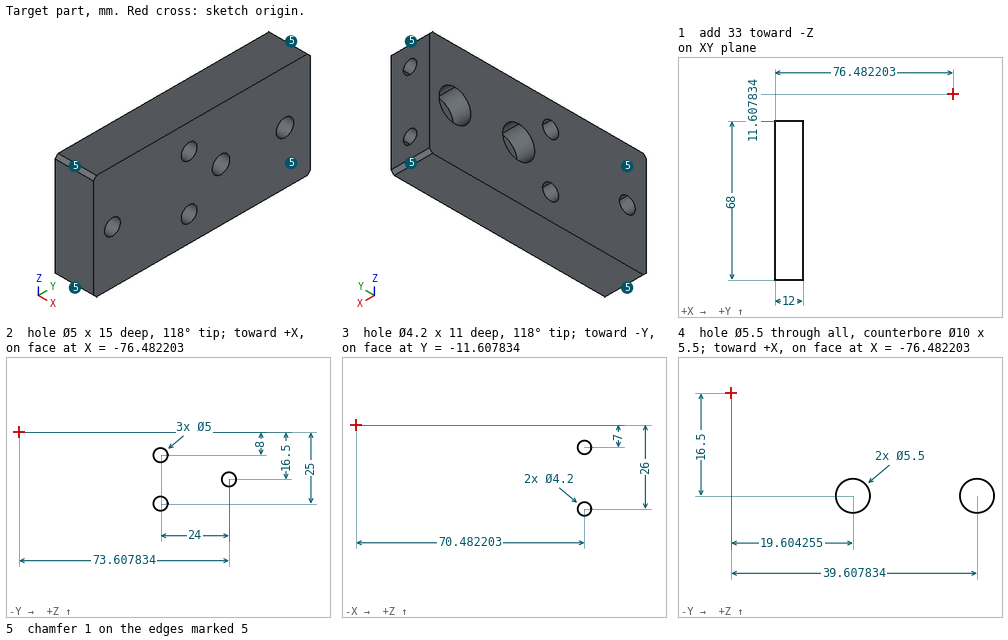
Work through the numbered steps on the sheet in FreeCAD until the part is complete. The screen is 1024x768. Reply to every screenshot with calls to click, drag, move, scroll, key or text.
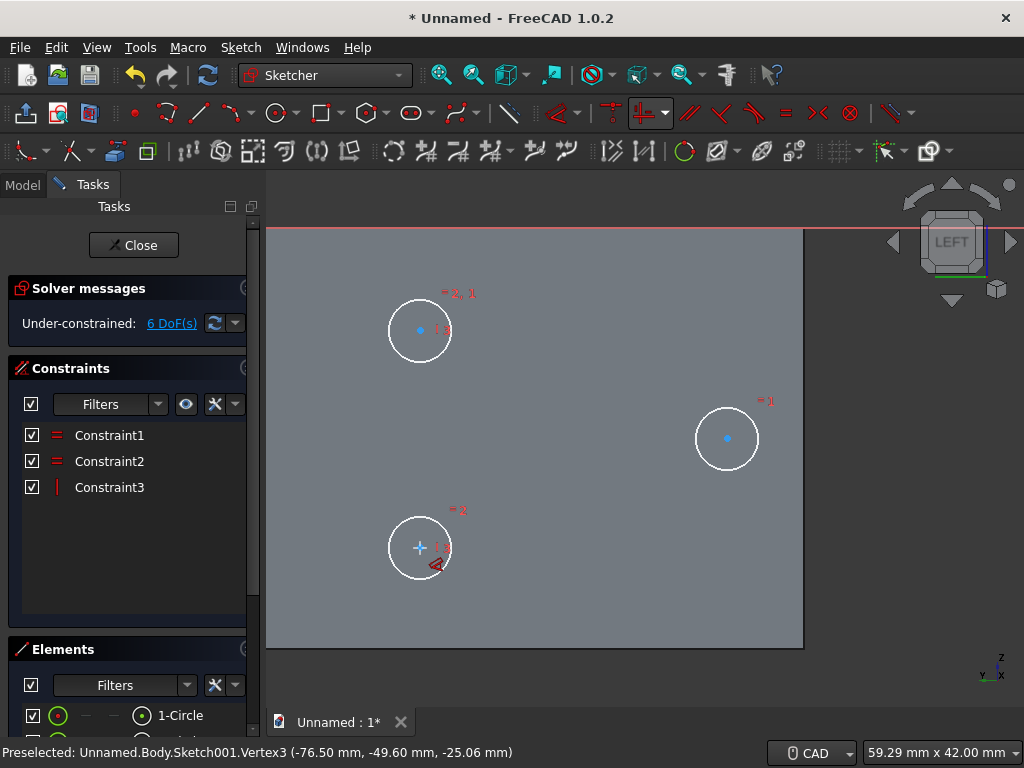
click(749, 417)
click(772, 394)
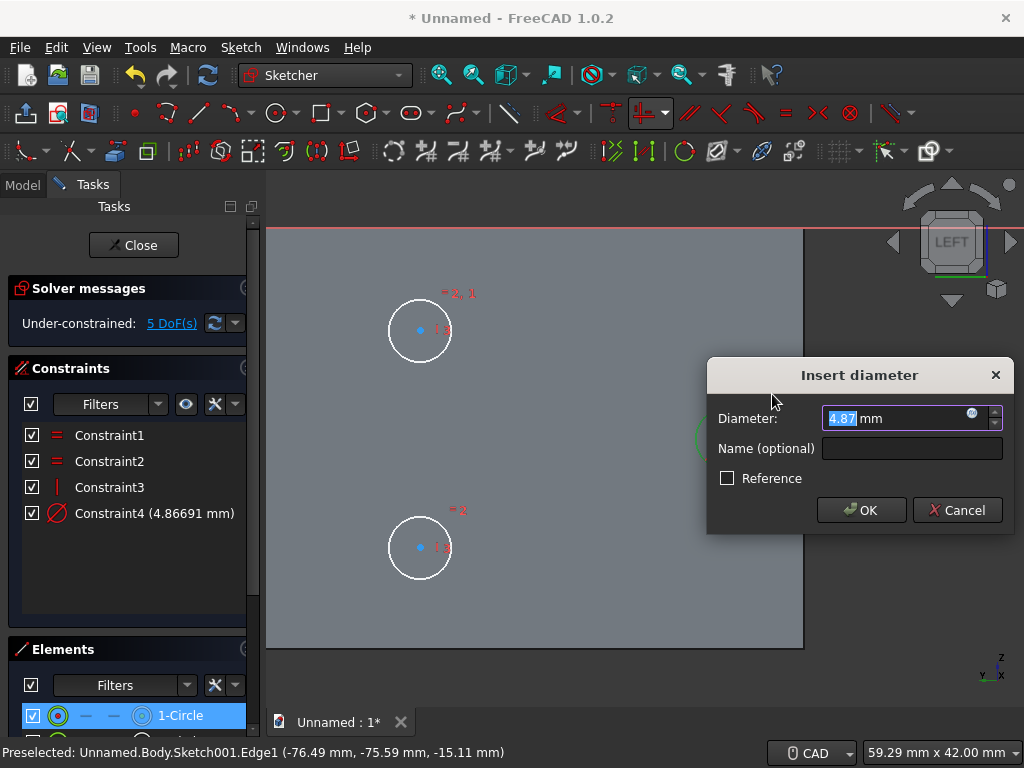
text(5)
key(Return)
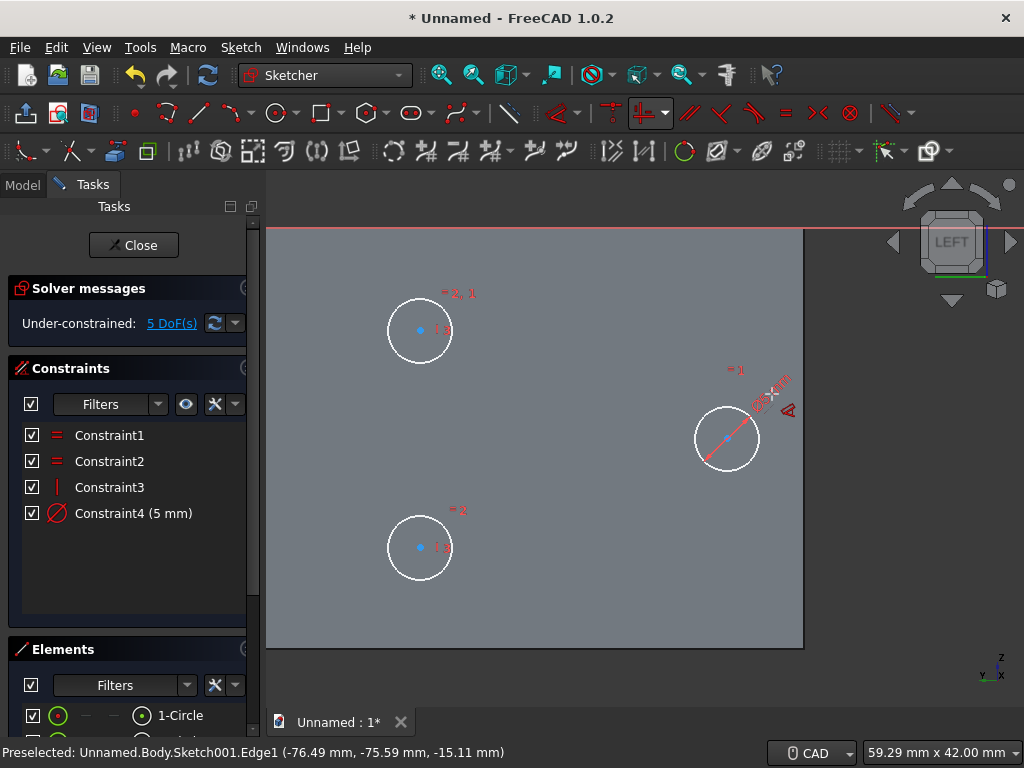
click(420, 331)
click(454, 279)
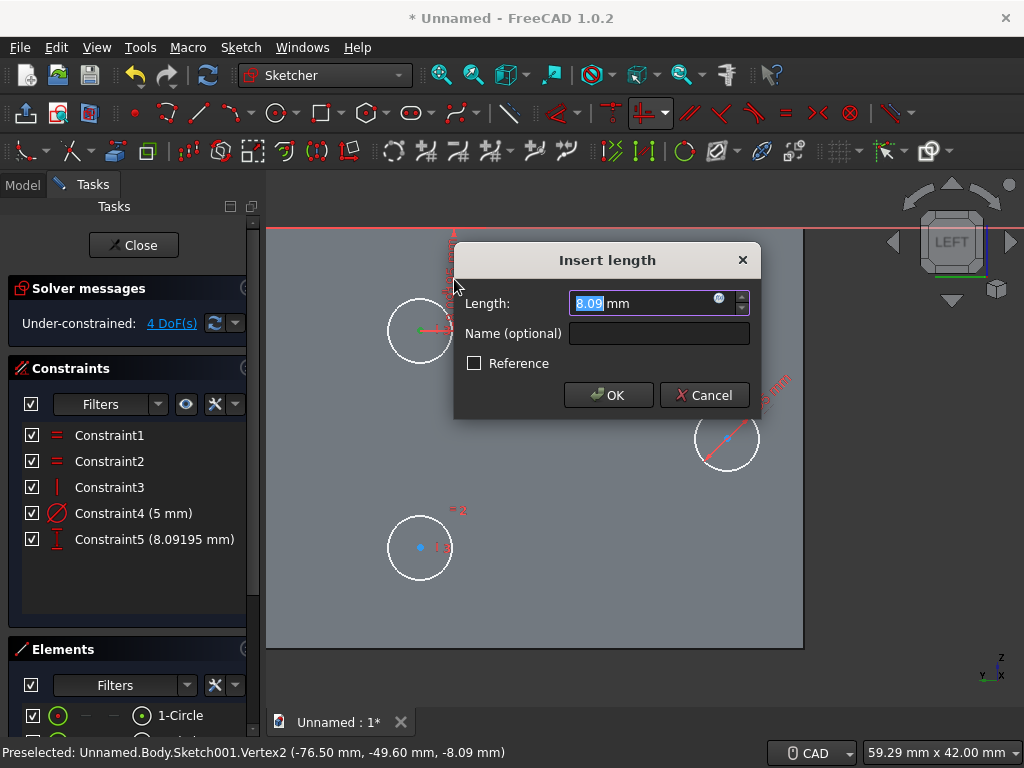
text(8)
key(Return)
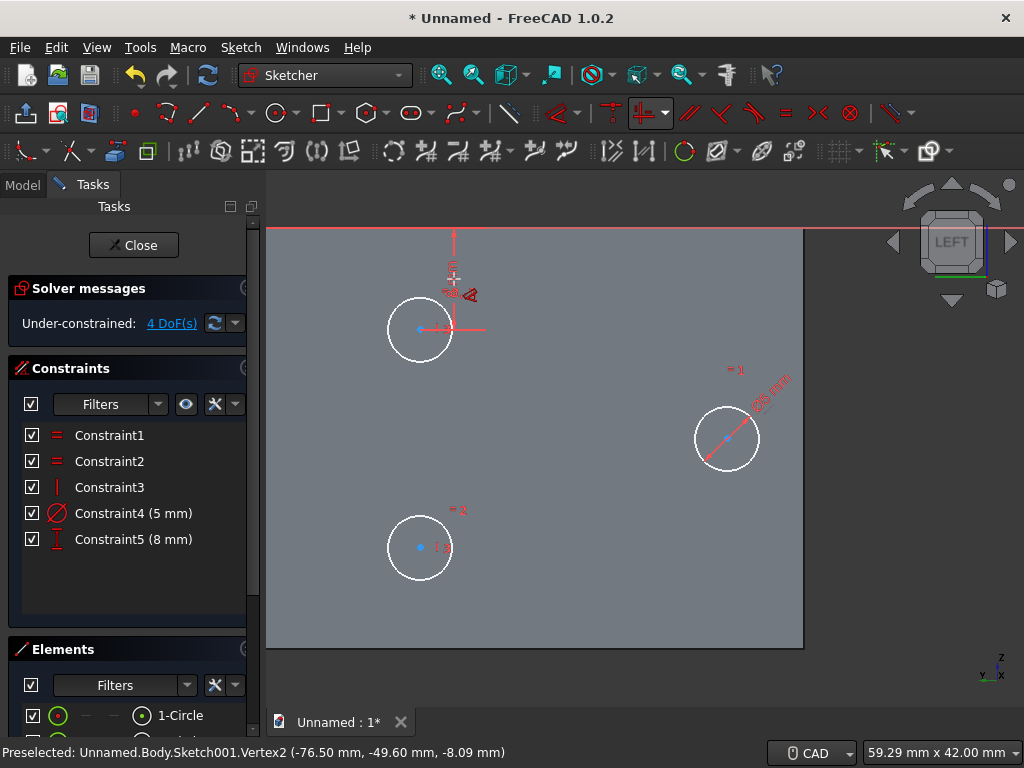
click(420, 548)
click(454, 388)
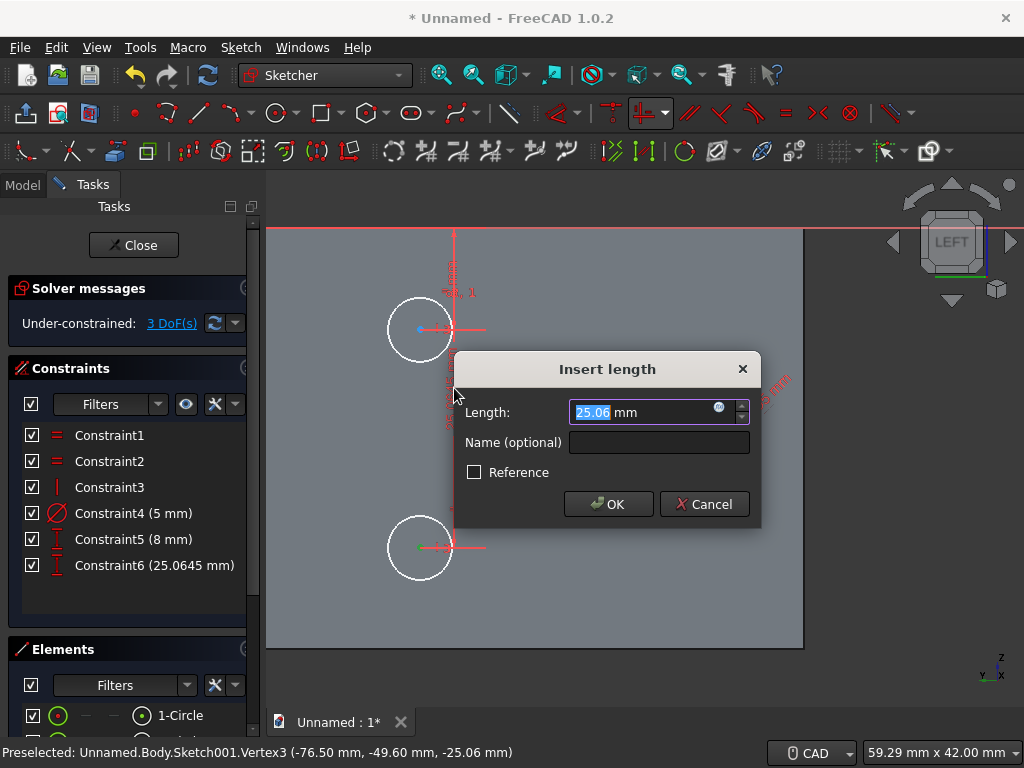
text(25)
key(Return)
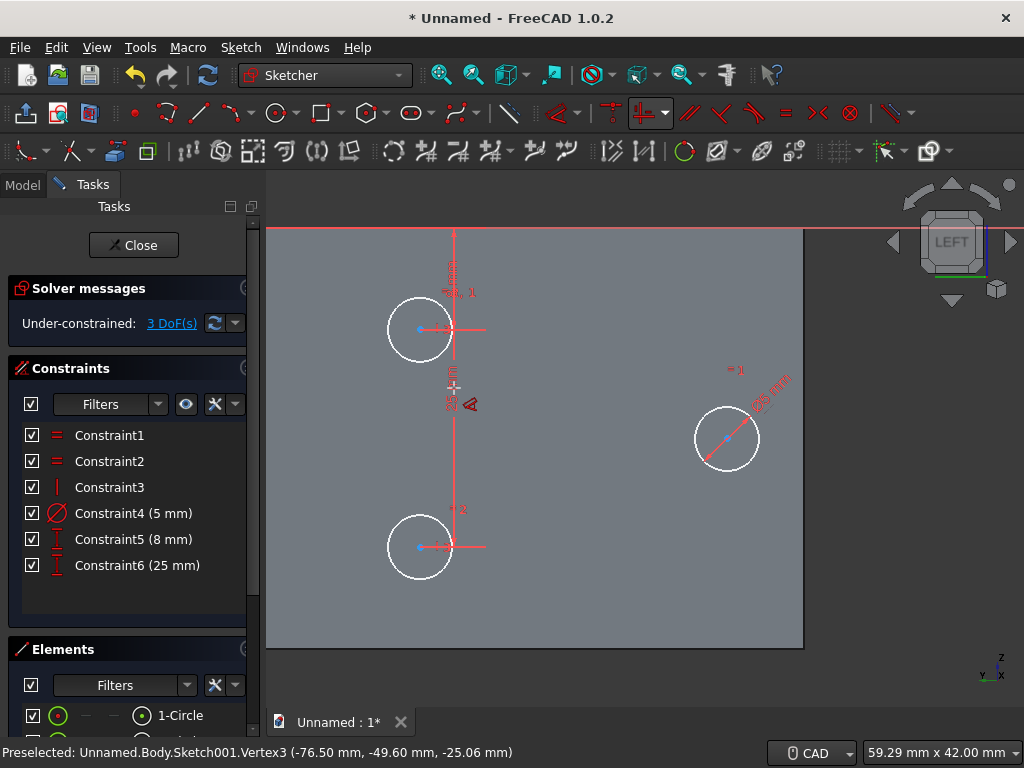
click(727, 439)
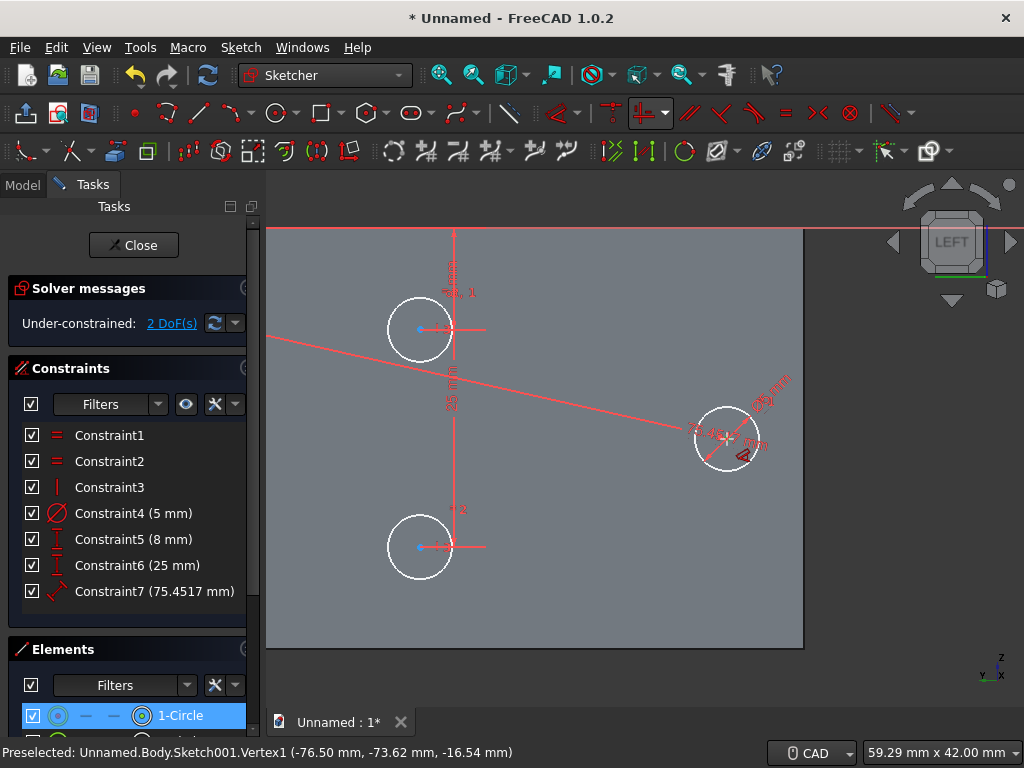
click(420, 330)
click(574, 296)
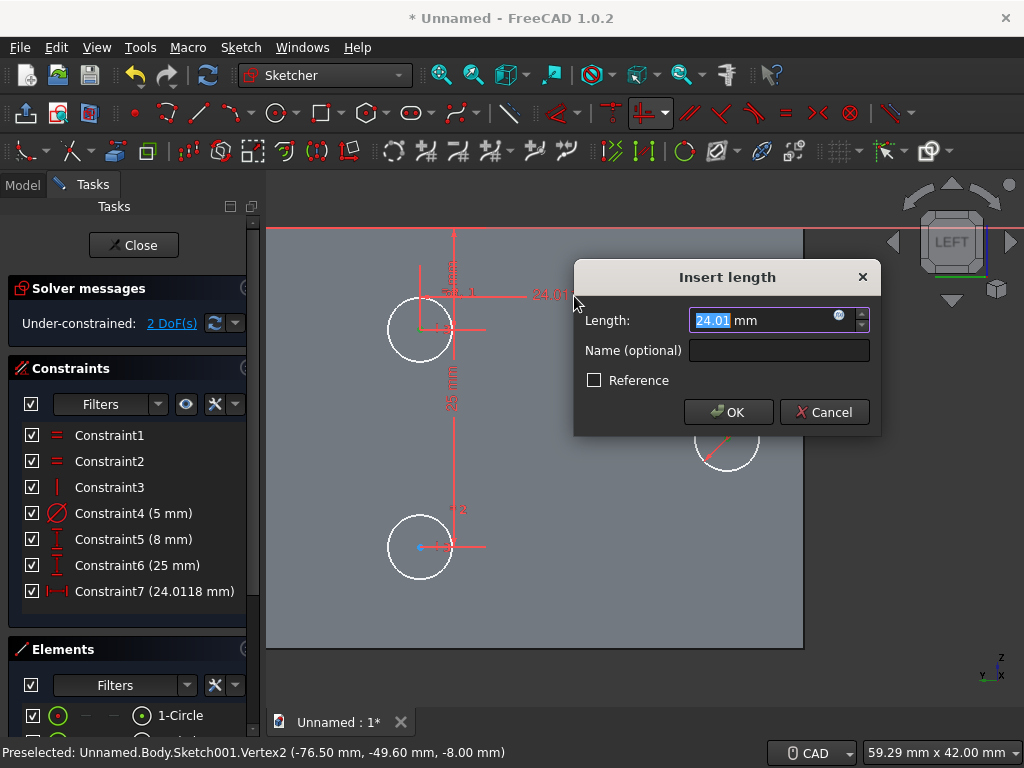
text(24)
key(Return)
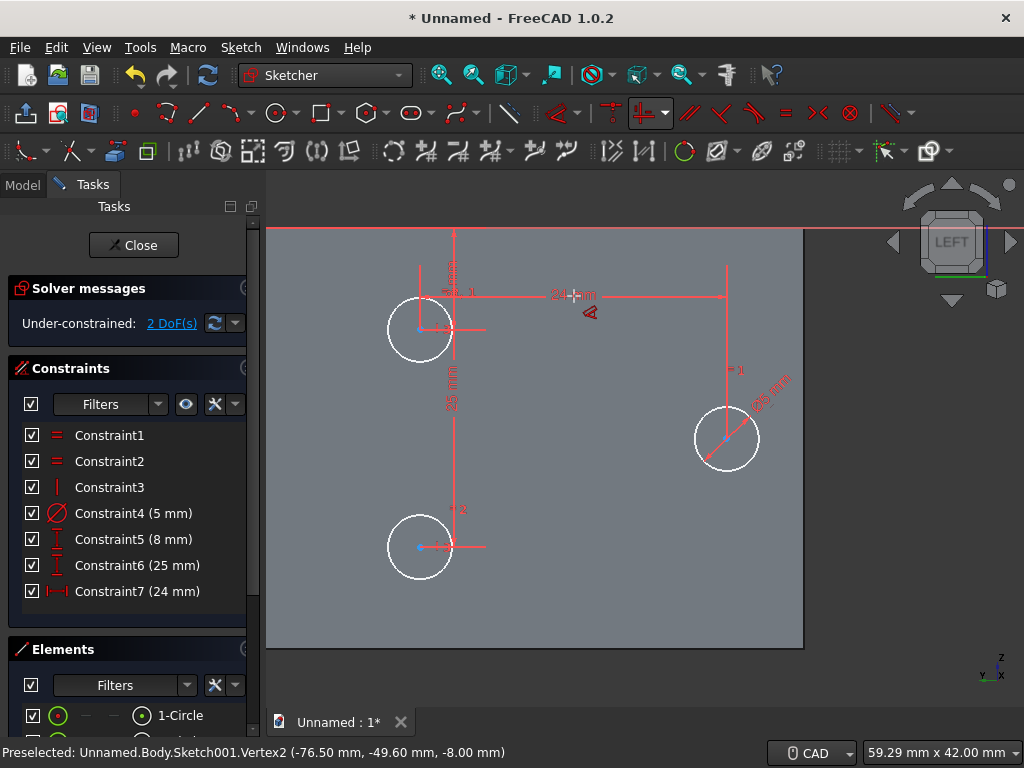
click(727, 439)
click(761, 333)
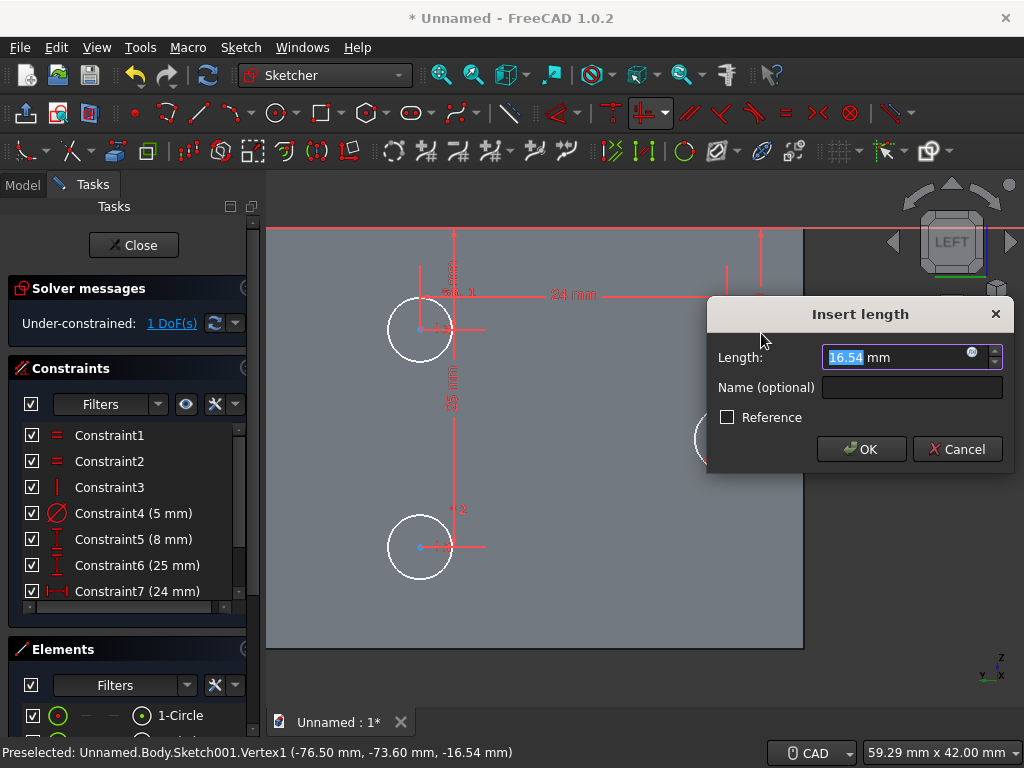
text(16.5)
key(Return)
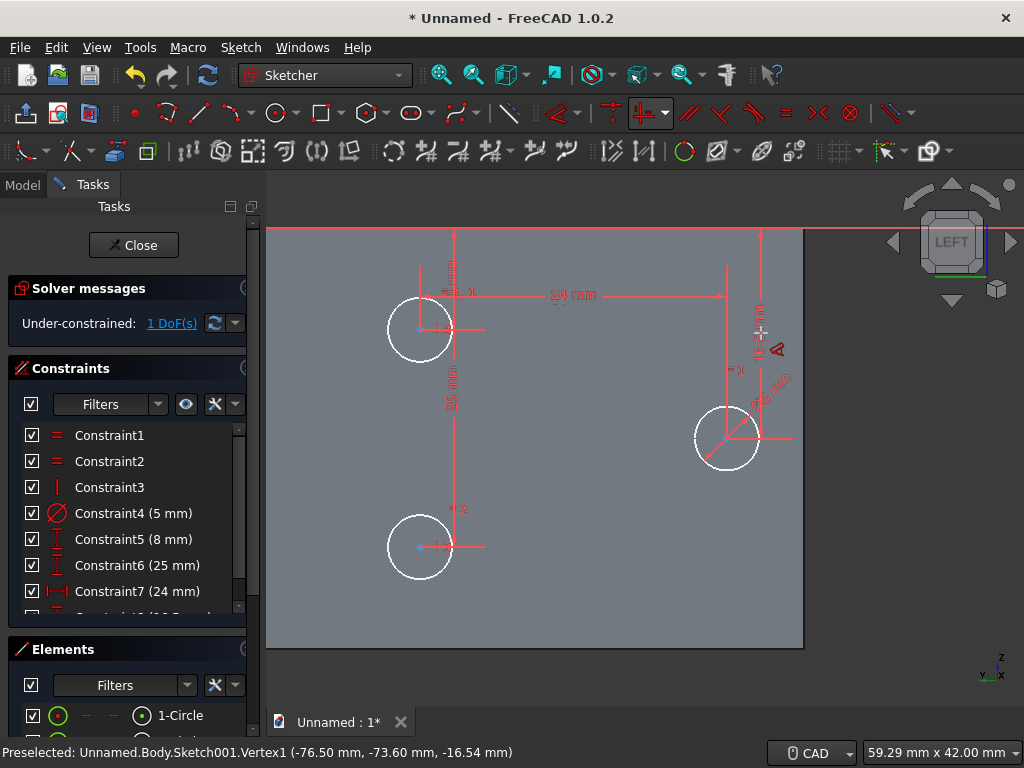
click(727, 438)
click(510, 472)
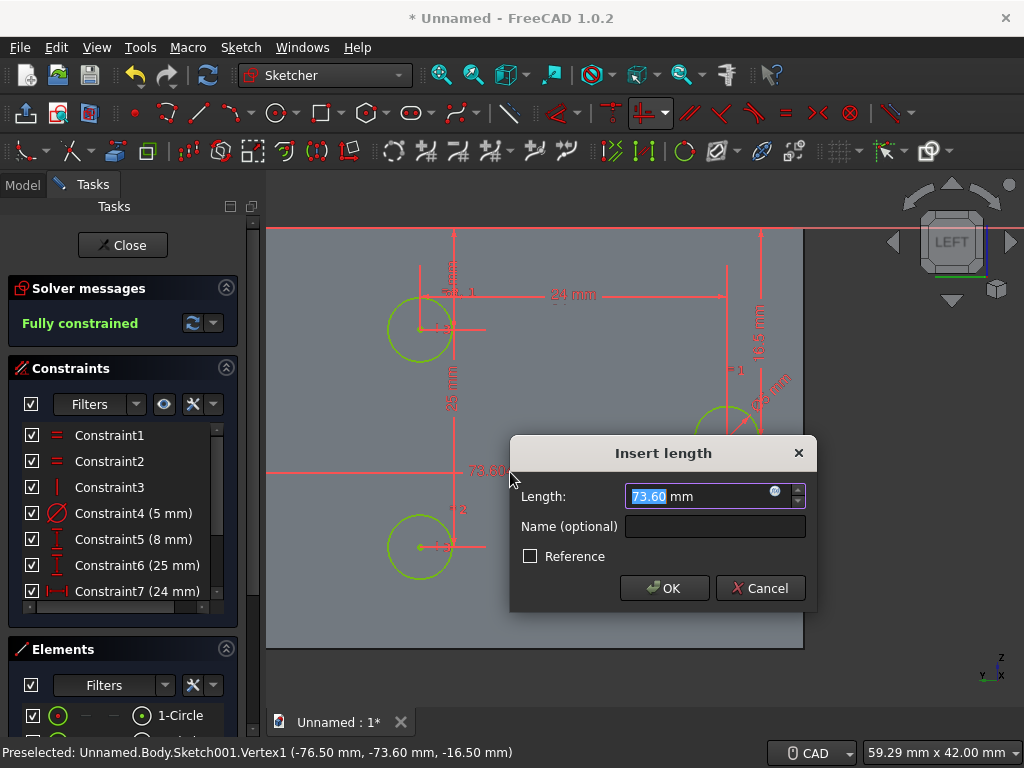
text(73.607834)
key(Return)
key(Escape)